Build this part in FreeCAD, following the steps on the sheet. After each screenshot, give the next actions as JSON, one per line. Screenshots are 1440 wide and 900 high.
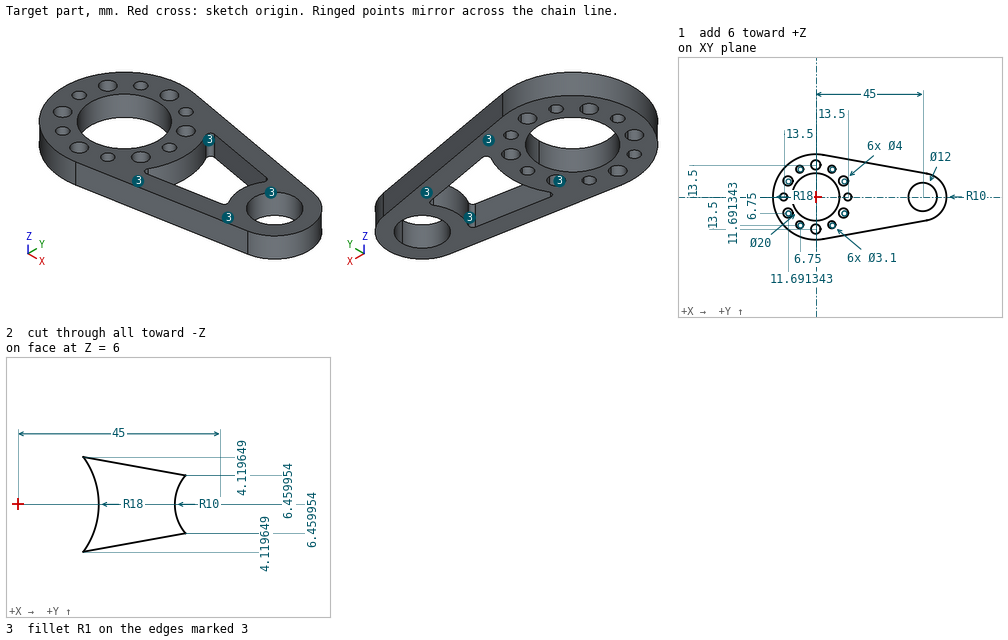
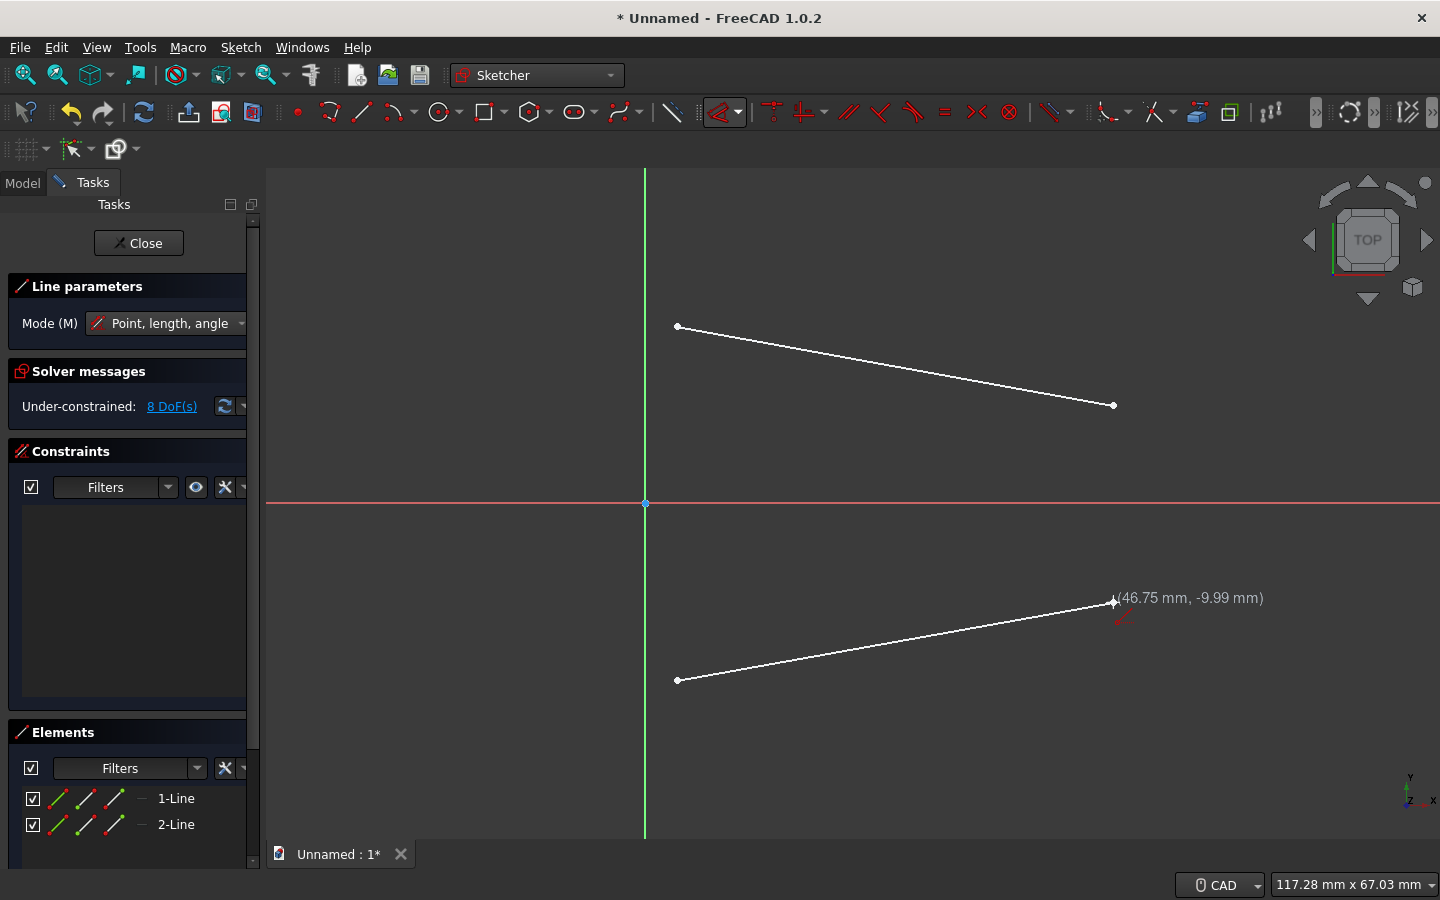
{"action": "key", "text": "g 3 a"}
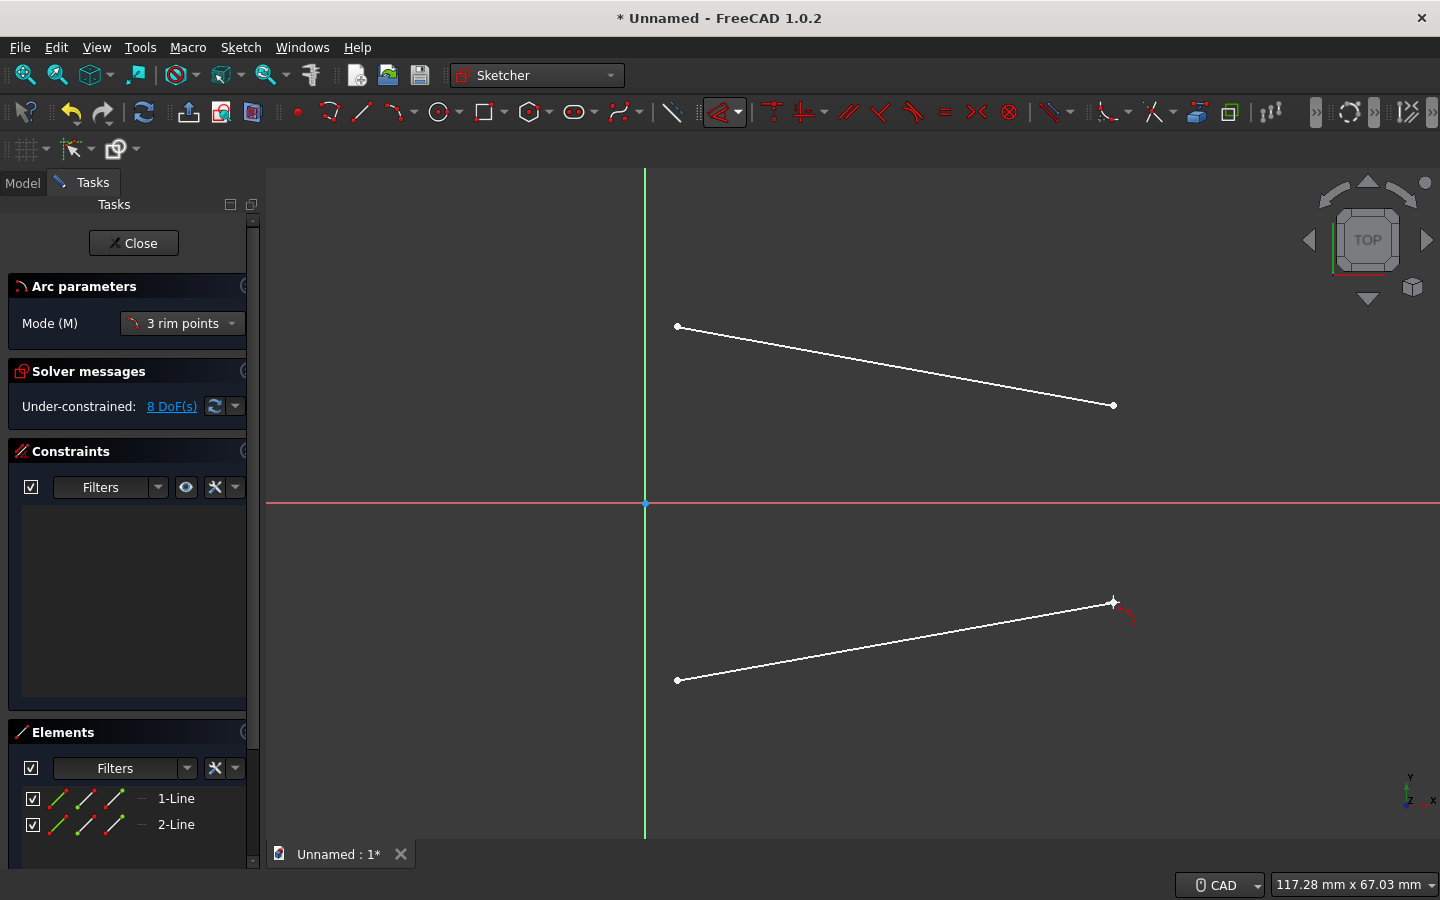
{"action": "left_click", "coordinate": [677, 327]}
{"action": "left_click", "coordinate": [677, 681]}
{"action": "left_click", "coordinate": [476, 441]}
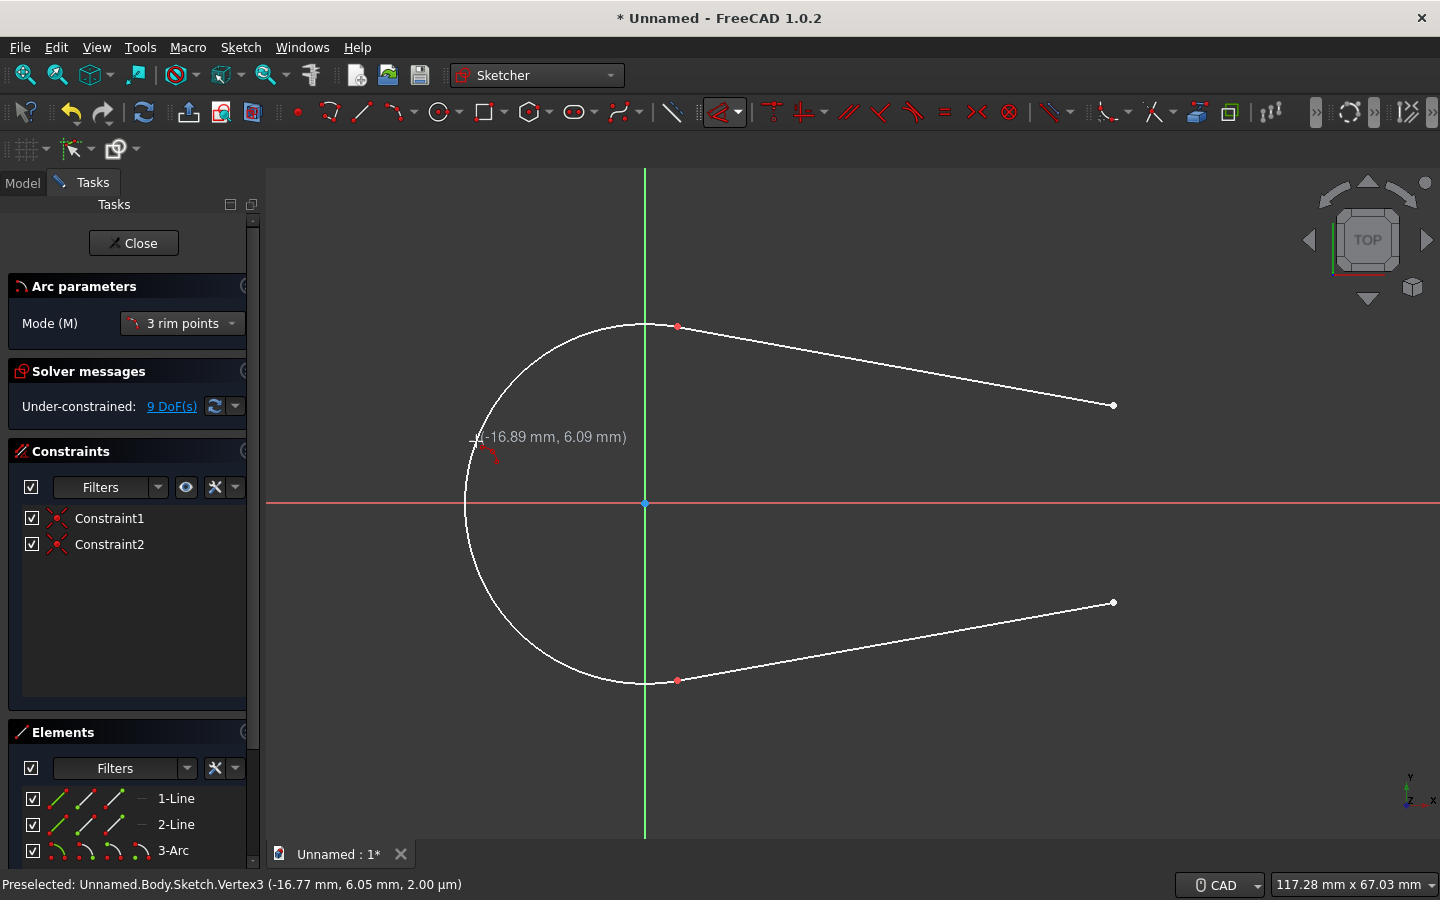
{"action": "left_click", "coordinate": [1113, 603]}
{"action": "left_click", "coordinate": [1113, 406]}
{"action": "left_click", "coordinate": [1192, 531]}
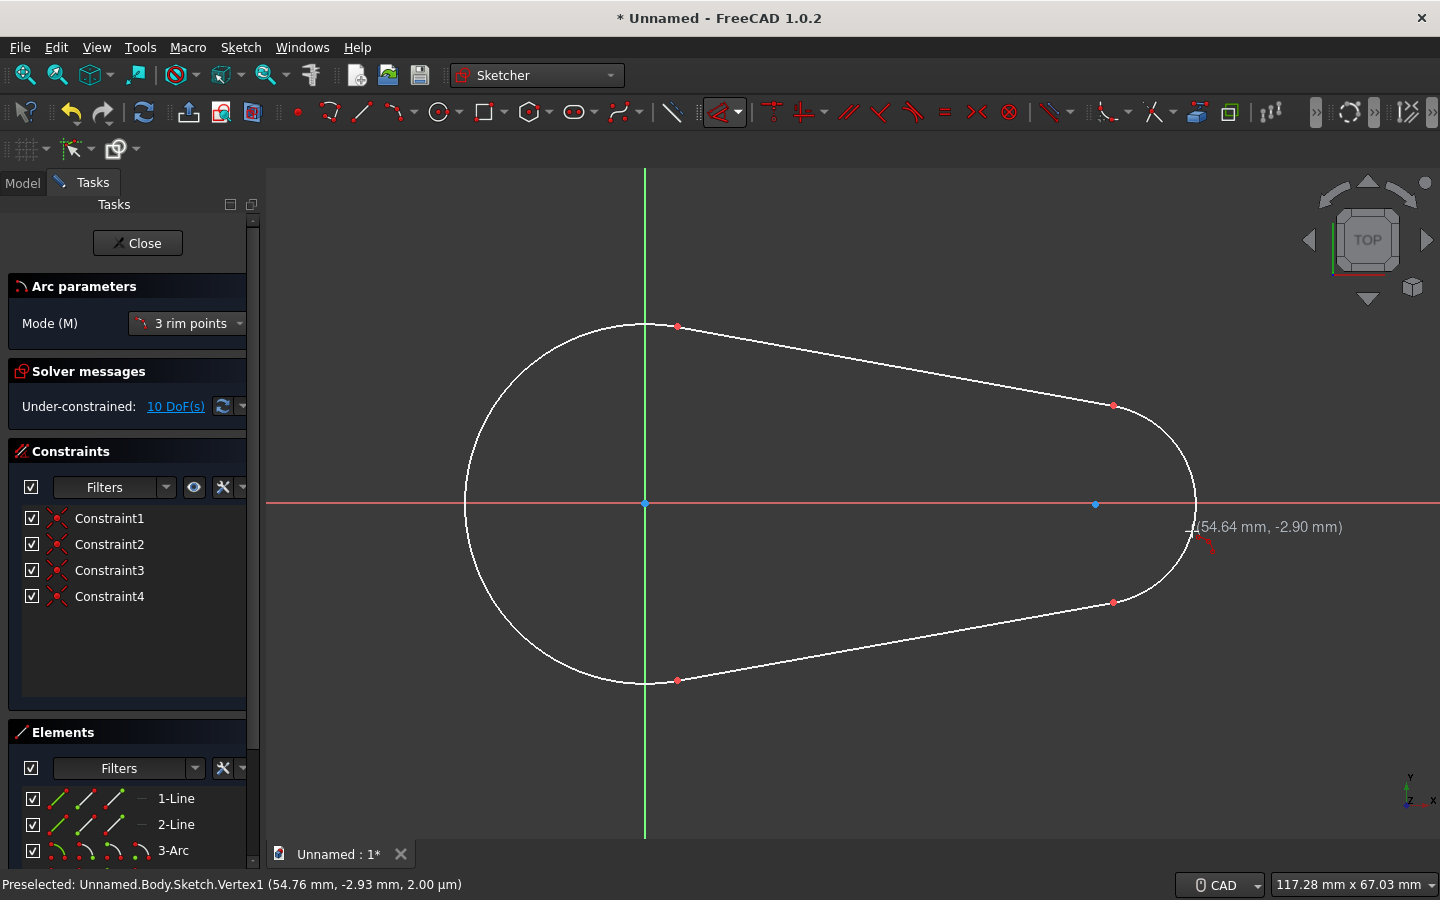
{"action": "key", "text": "g c"}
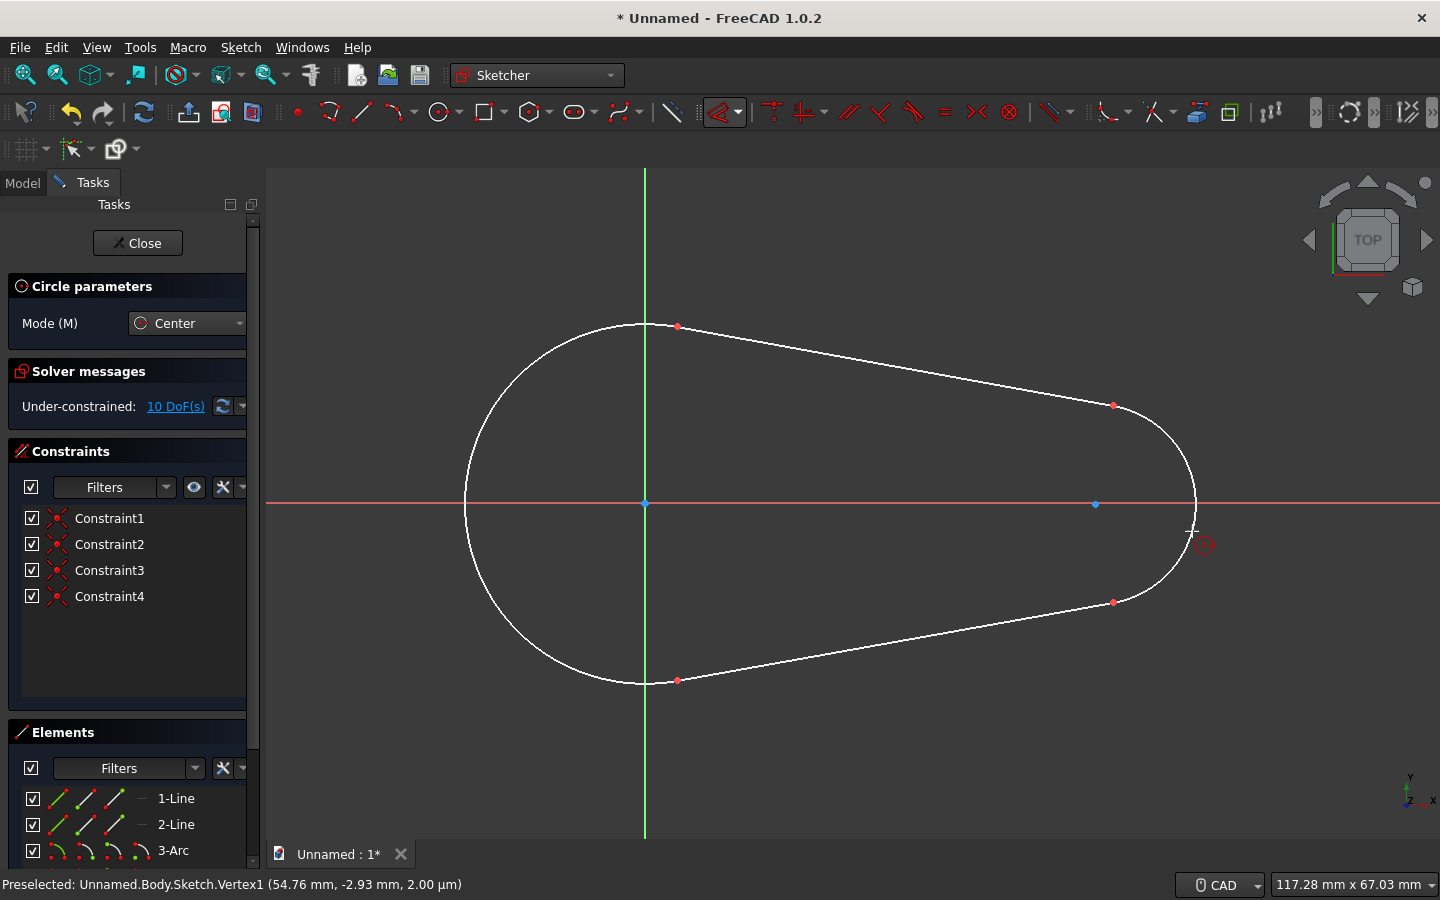
{"action": "scroll", "coordinate": [577, 620], "scroll_direction": "up", "scroll_amount": 2}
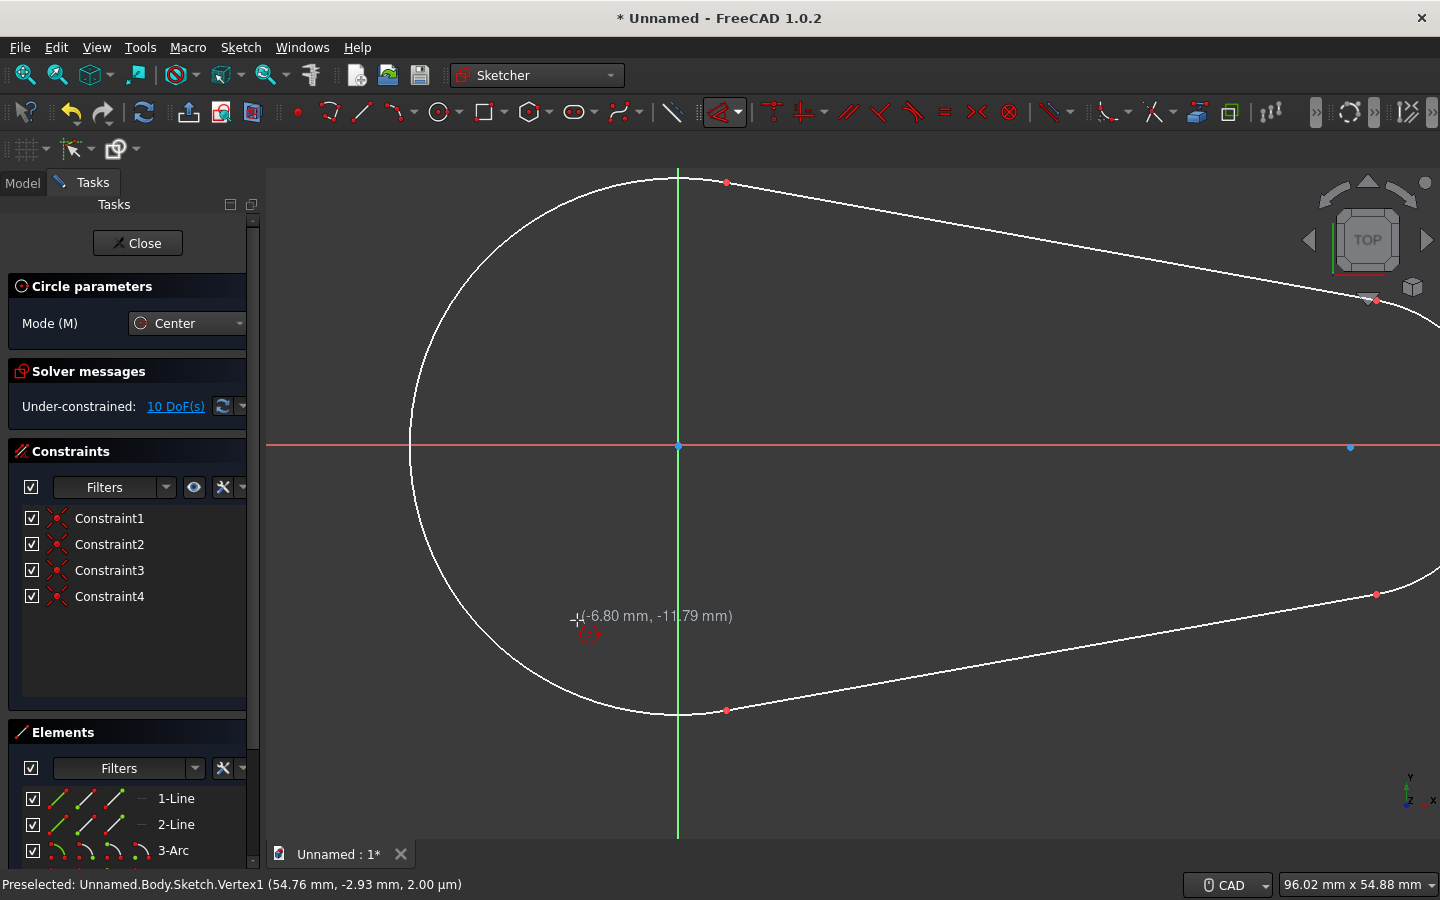
{"action": "left_click", "coordinate": [578, 620]}
{"action": "left_click", "coordinate": [594, 603]}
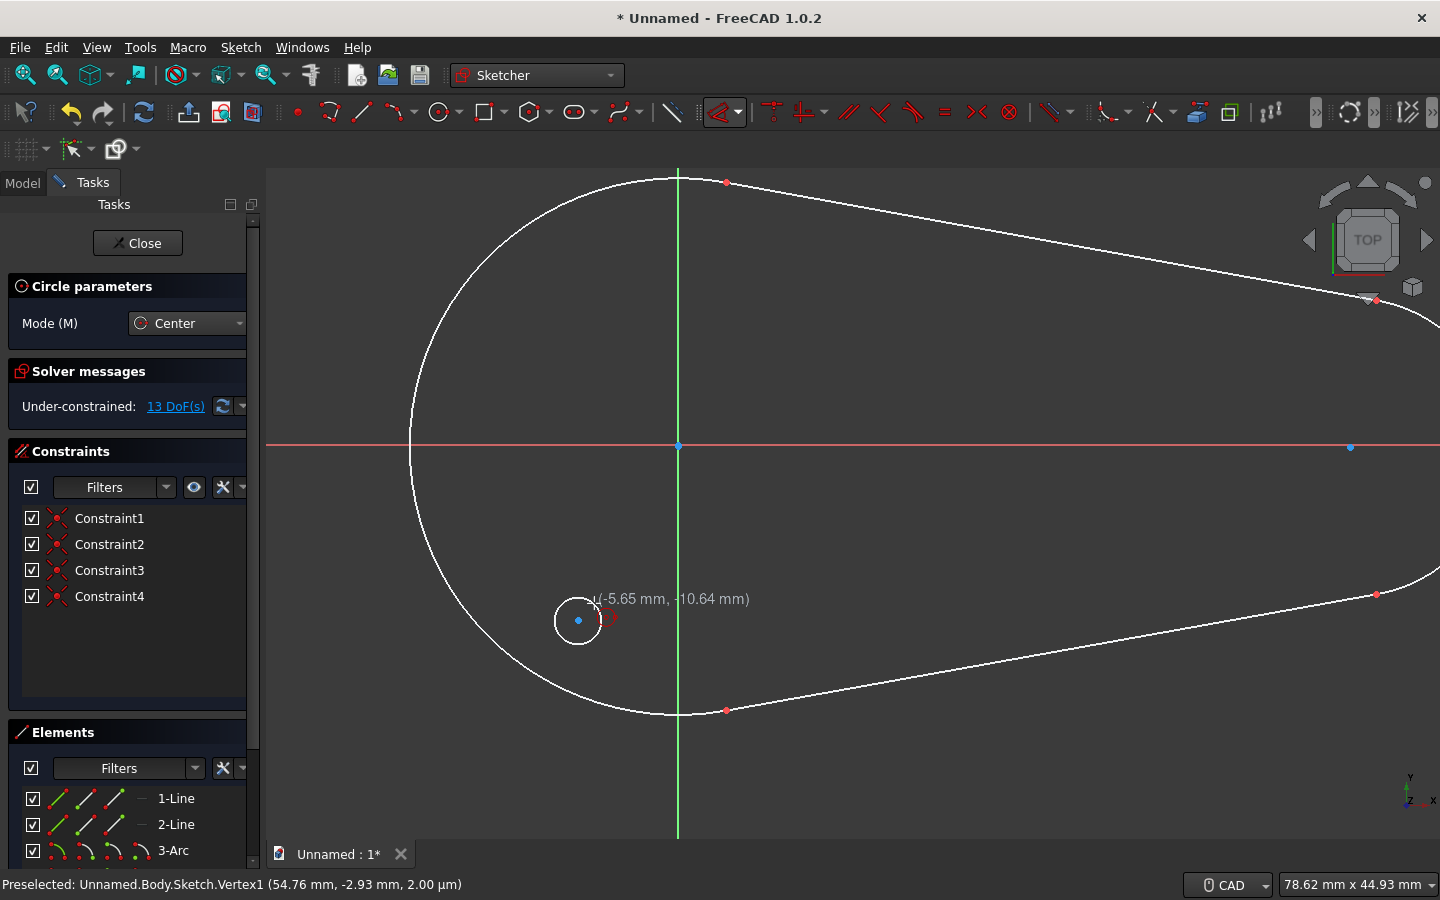
{"action": "left_click", "coordinate": [678, 647]}
{"action": "left_click", "coordinate": [699, 626]}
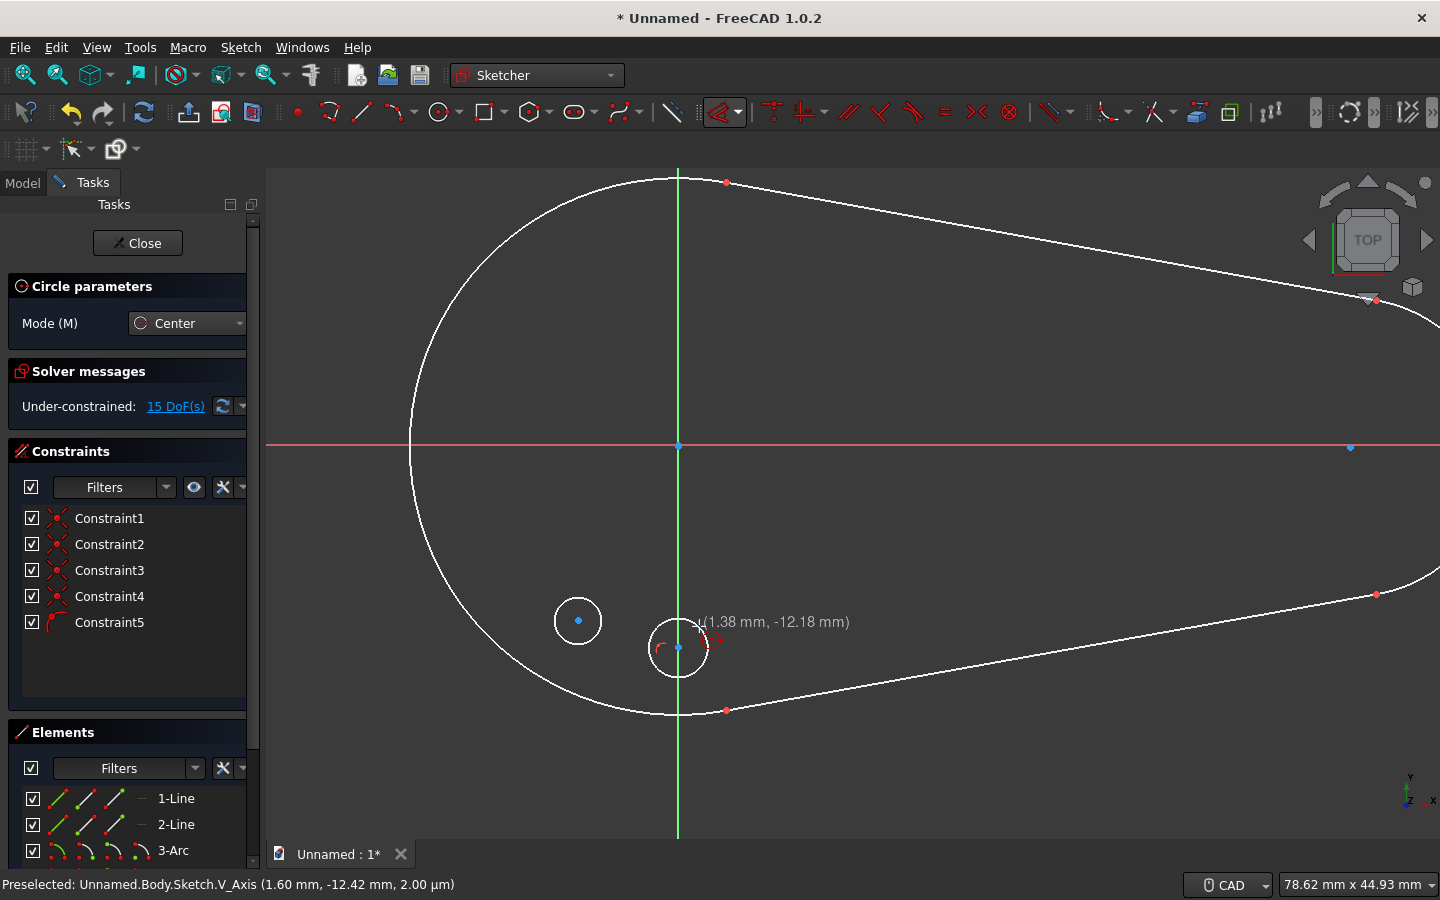
{"action": "left_click", "coordinate": [779, 620]}
{"action": "left_click", "coordinate": [796, 603]}